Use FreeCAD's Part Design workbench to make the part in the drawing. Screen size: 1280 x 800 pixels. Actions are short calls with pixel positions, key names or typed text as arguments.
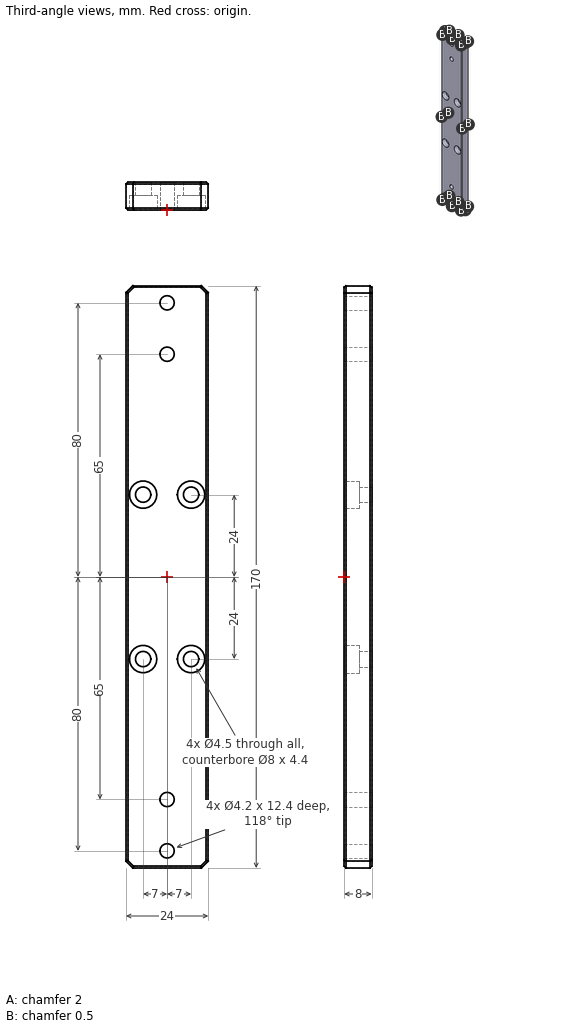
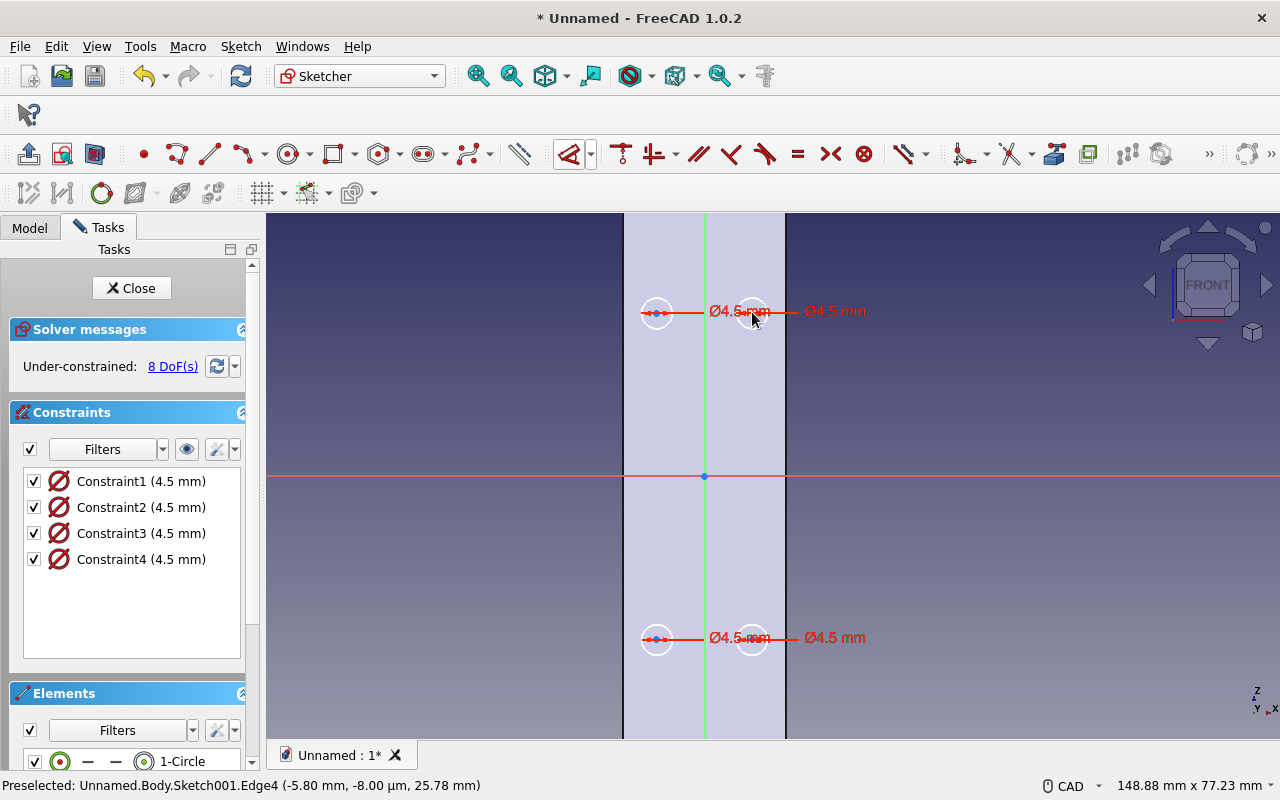
click(752, 640)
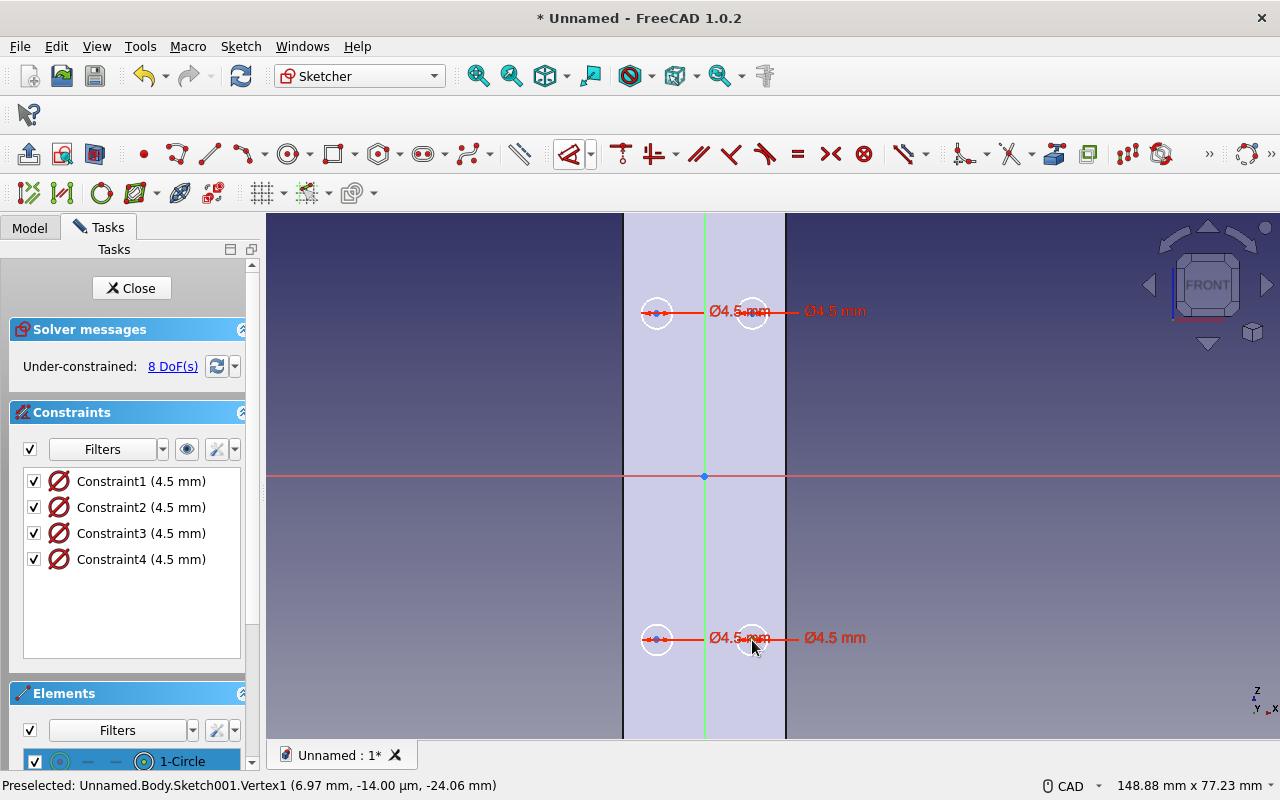
click(657, 640)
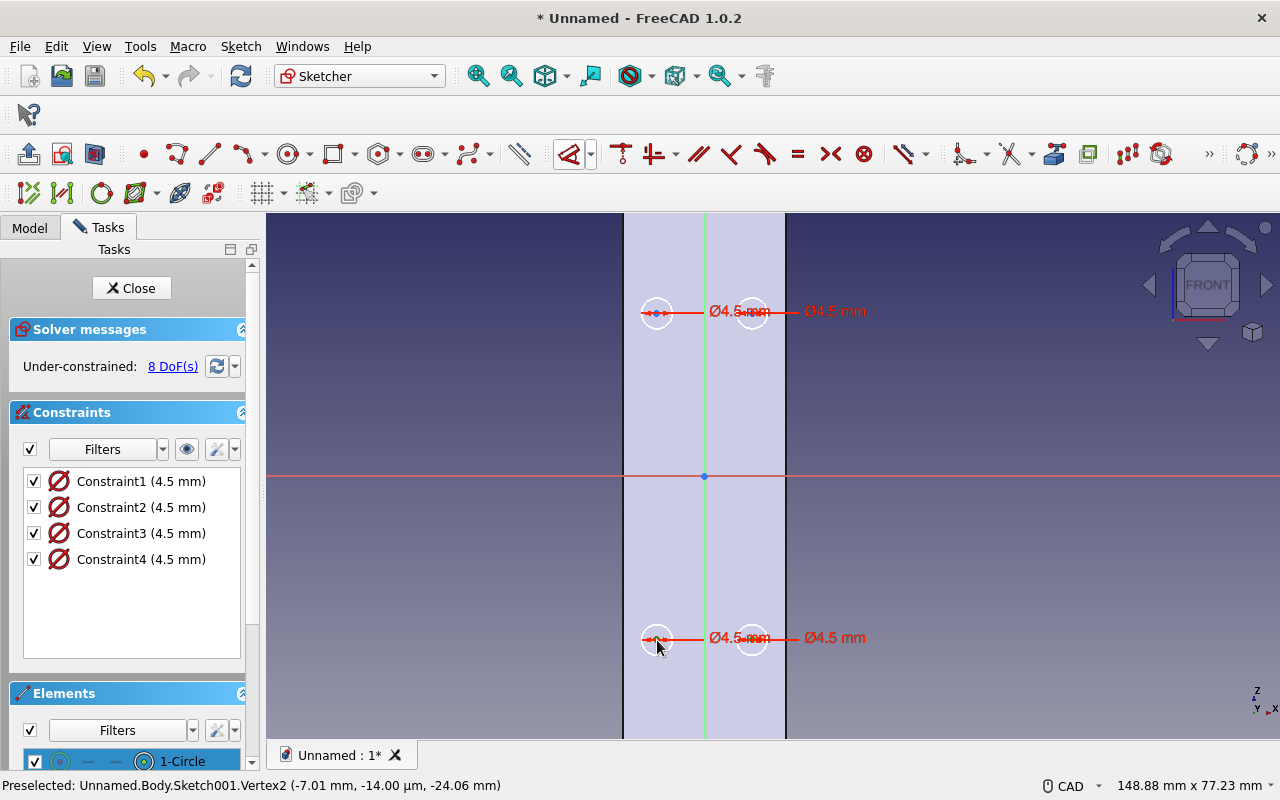
click(676, 154)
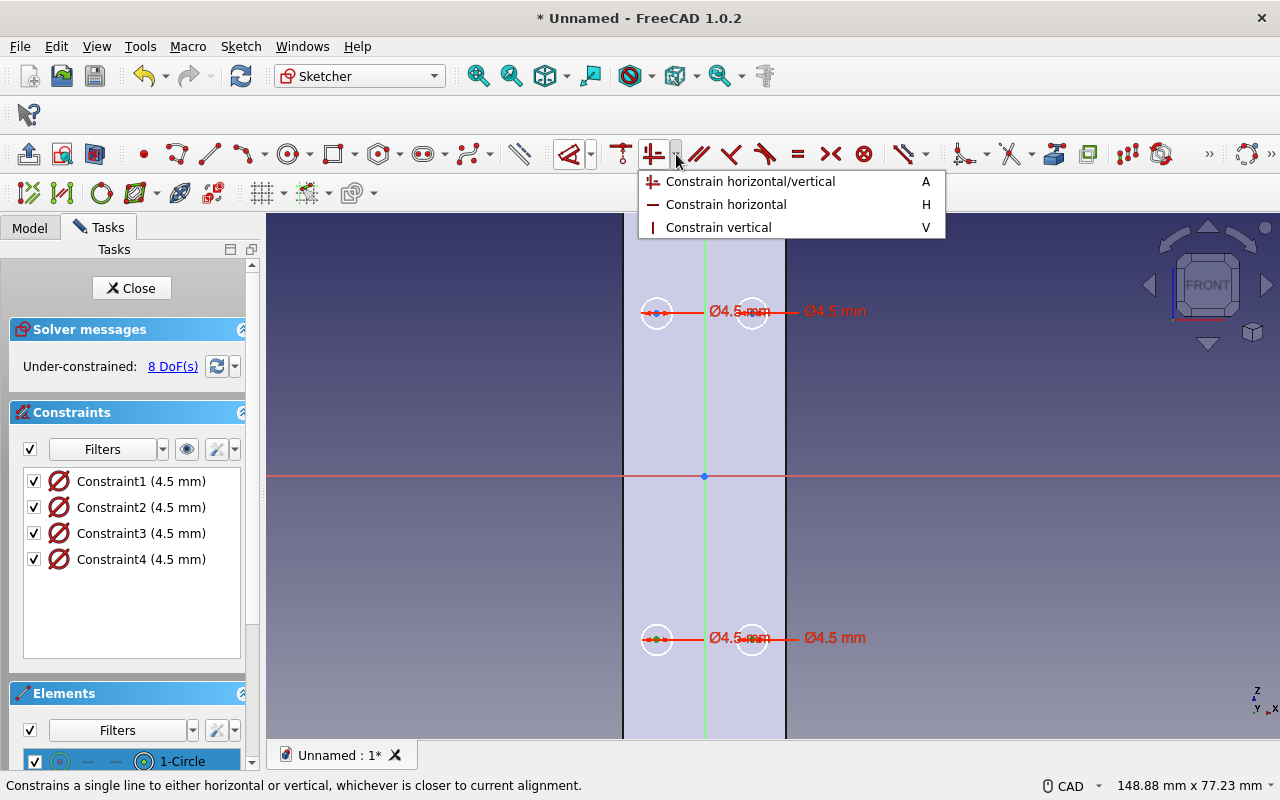
click(792, 204)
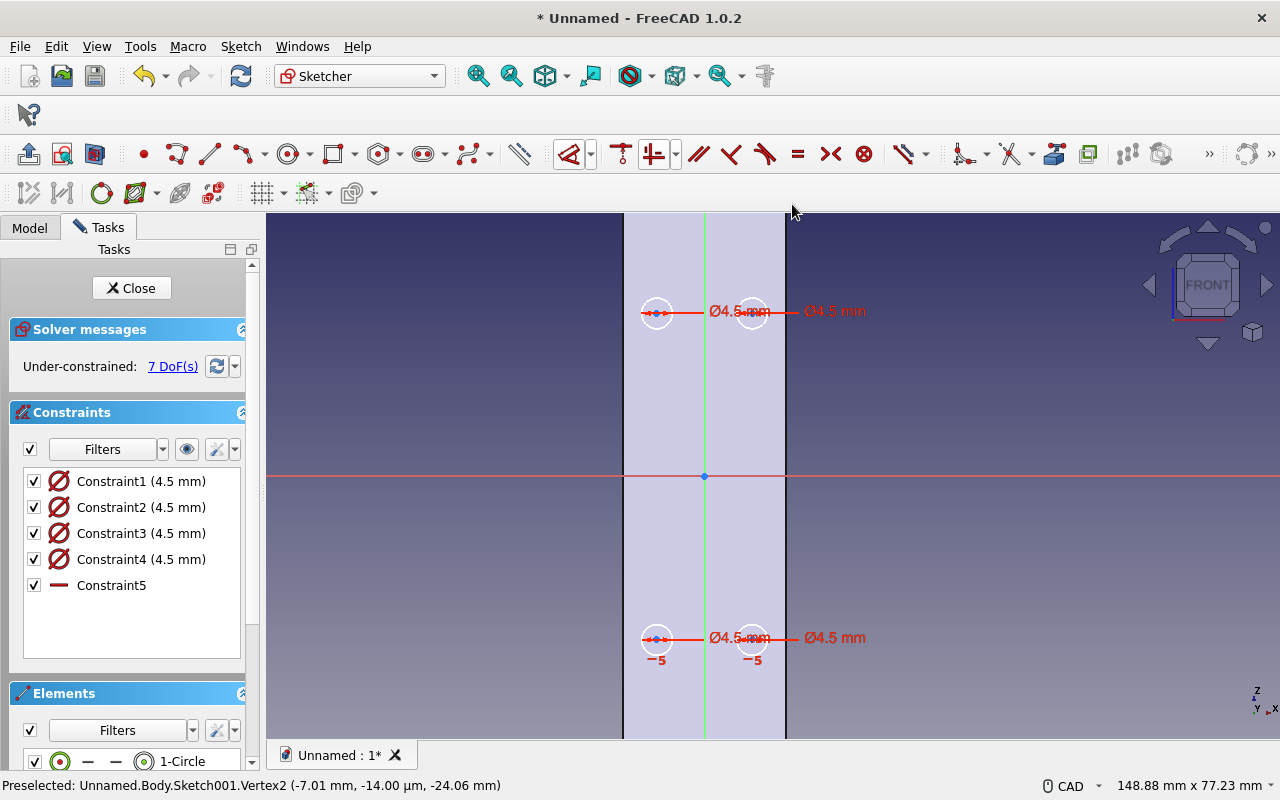
click(752, 640)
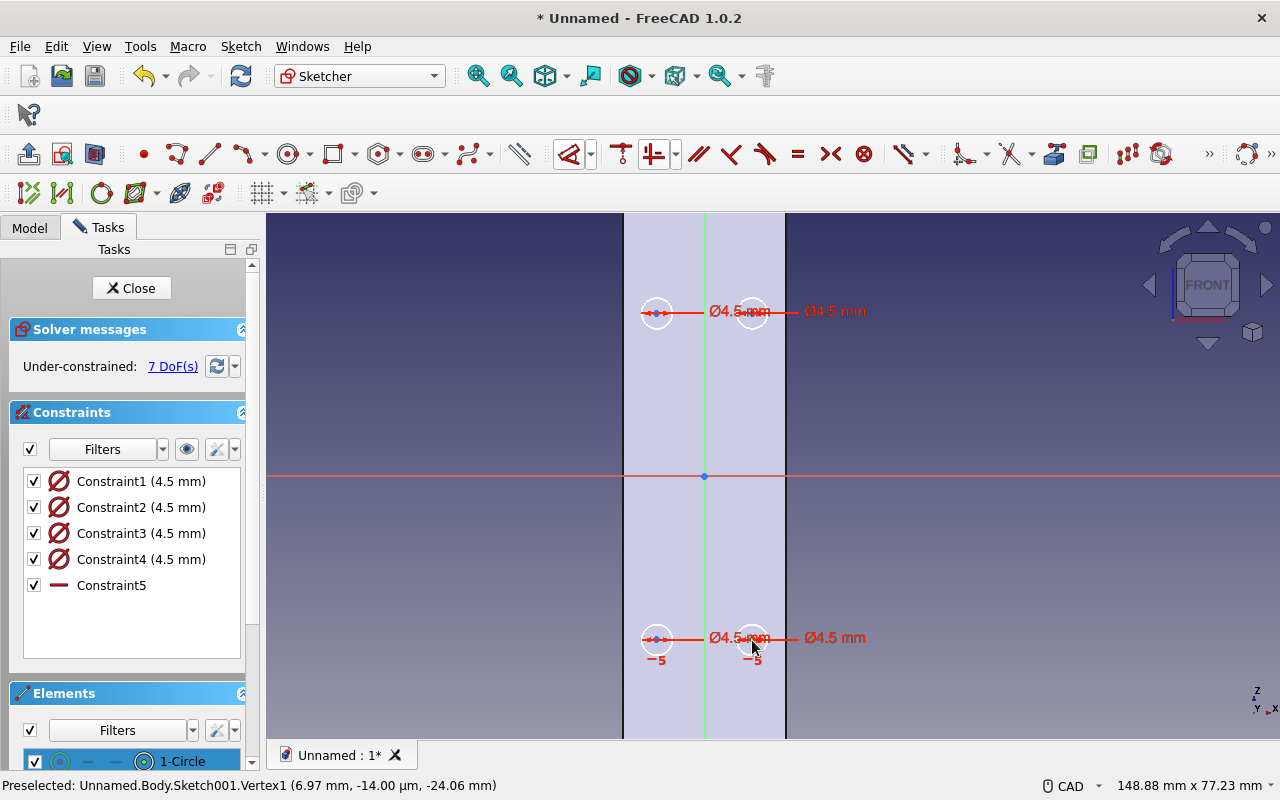
click(752, 313)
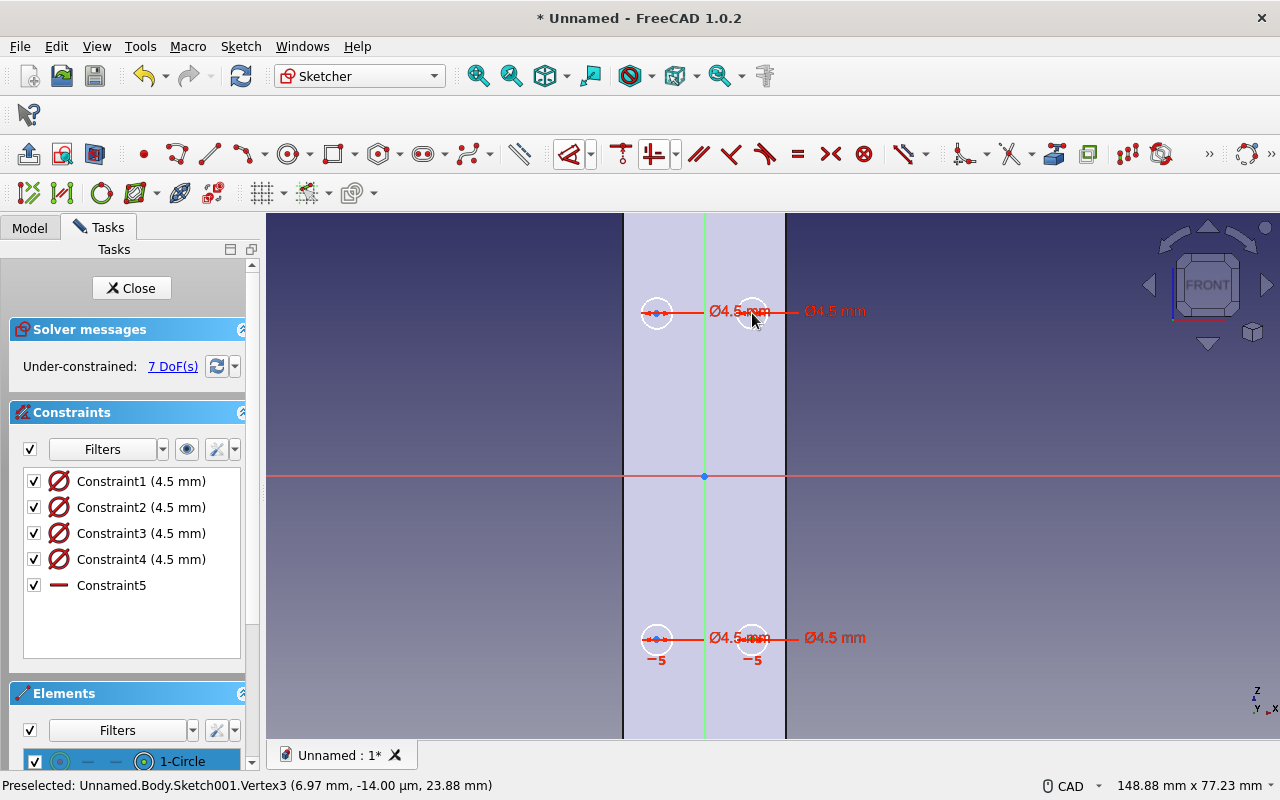
click(676, 154)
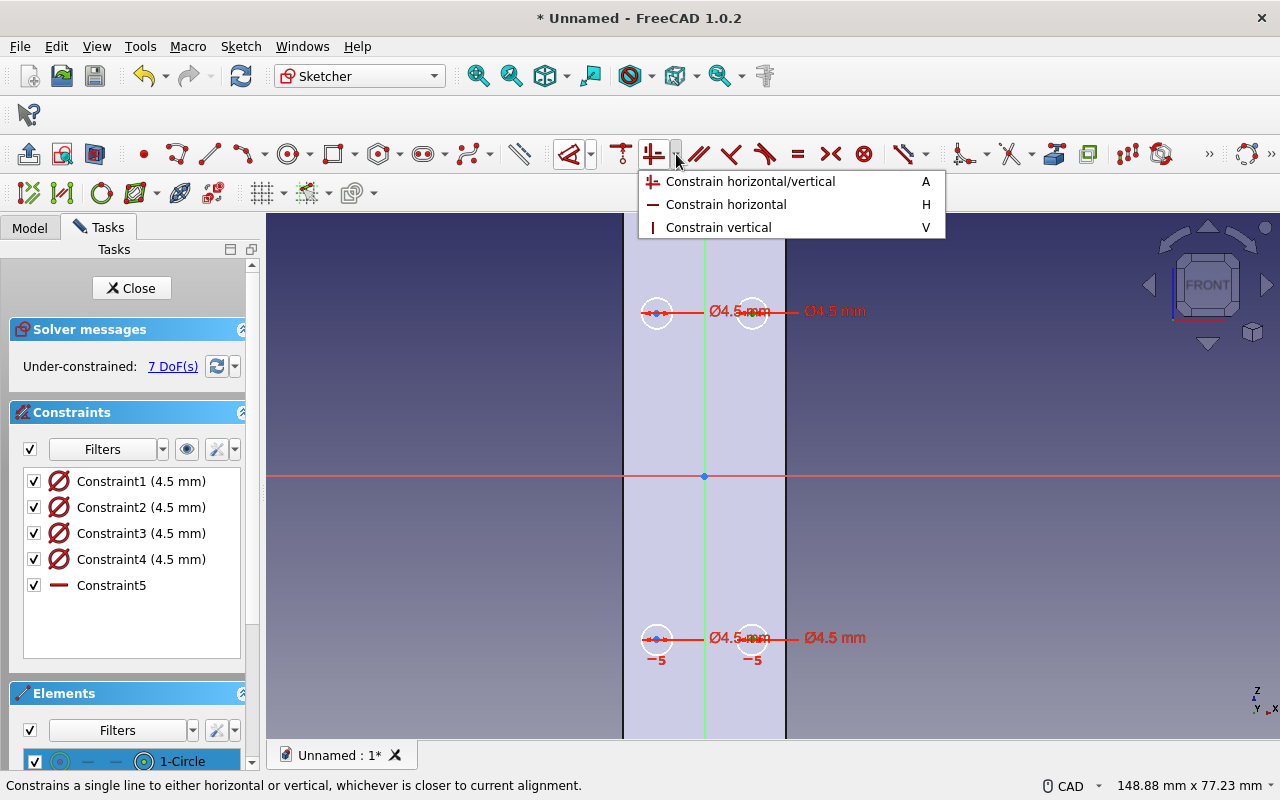
click(792, 228)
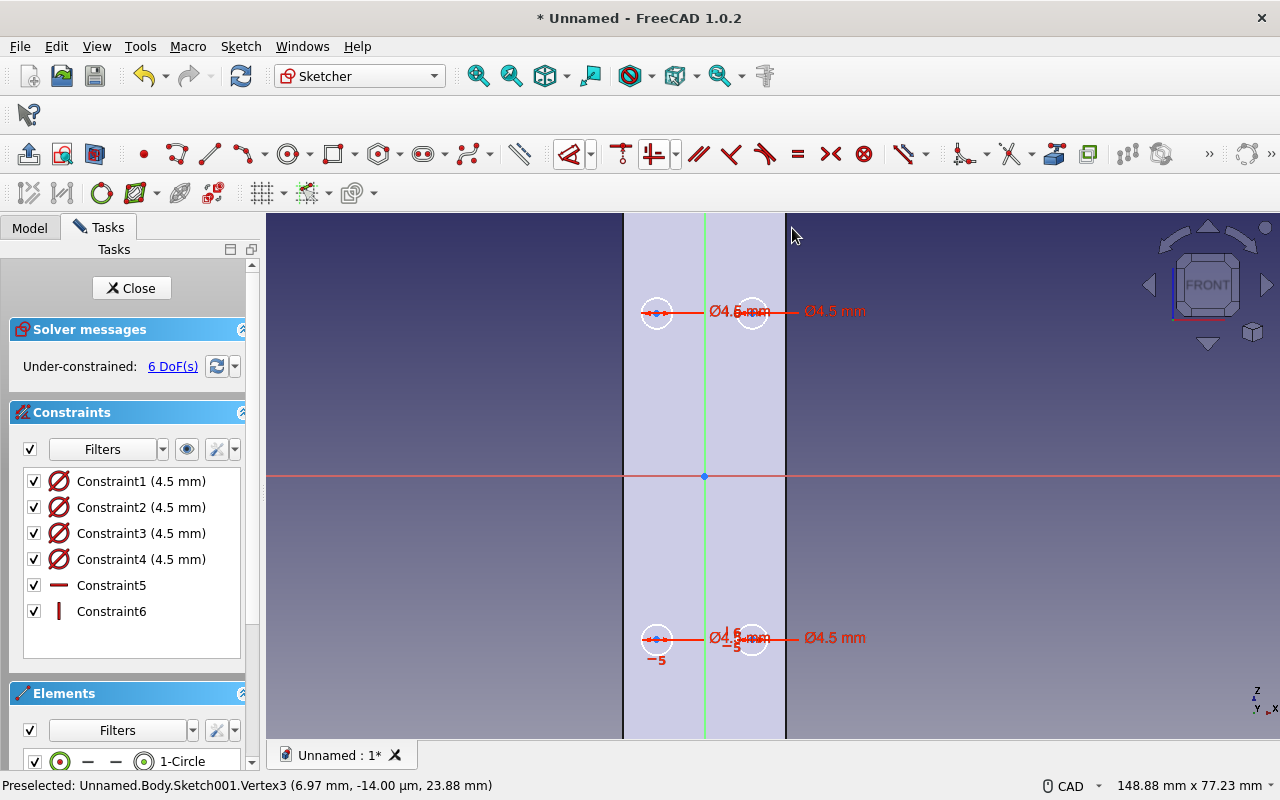
click(657, 640)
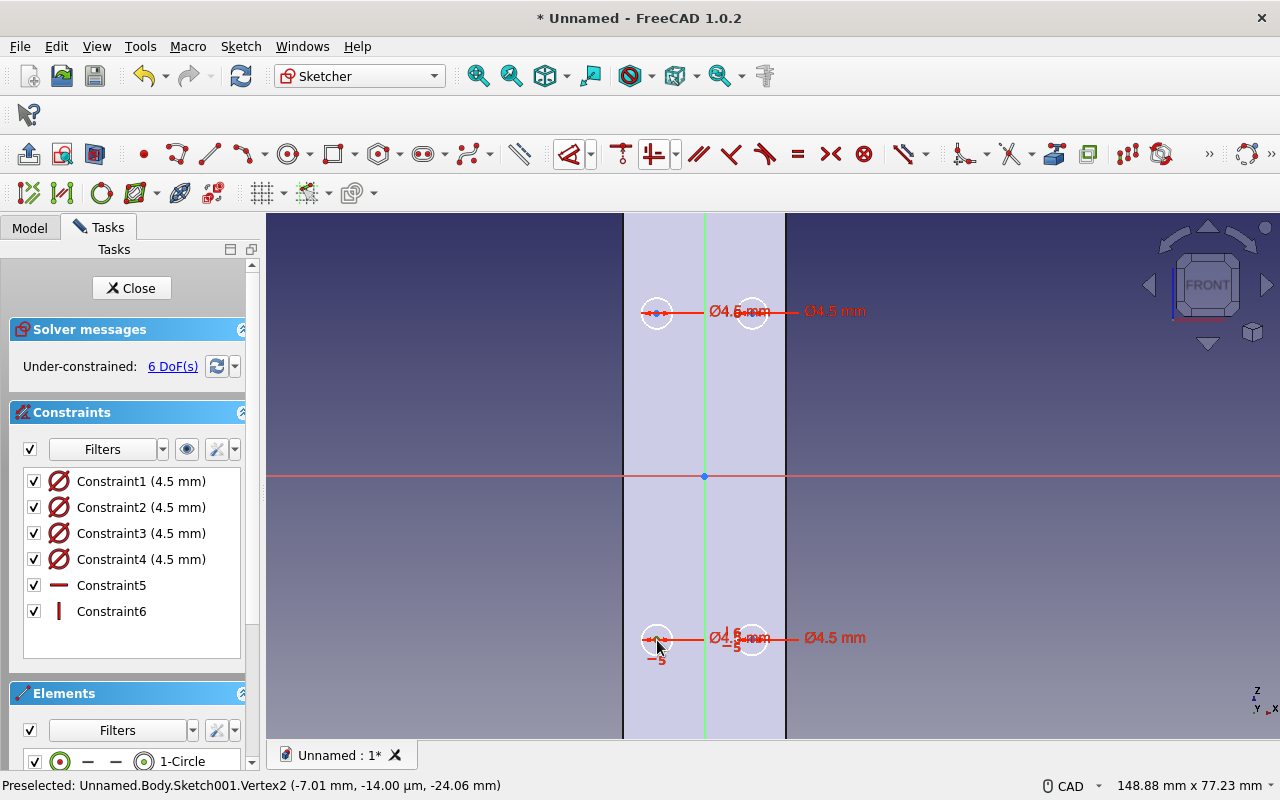
click(657, 313)